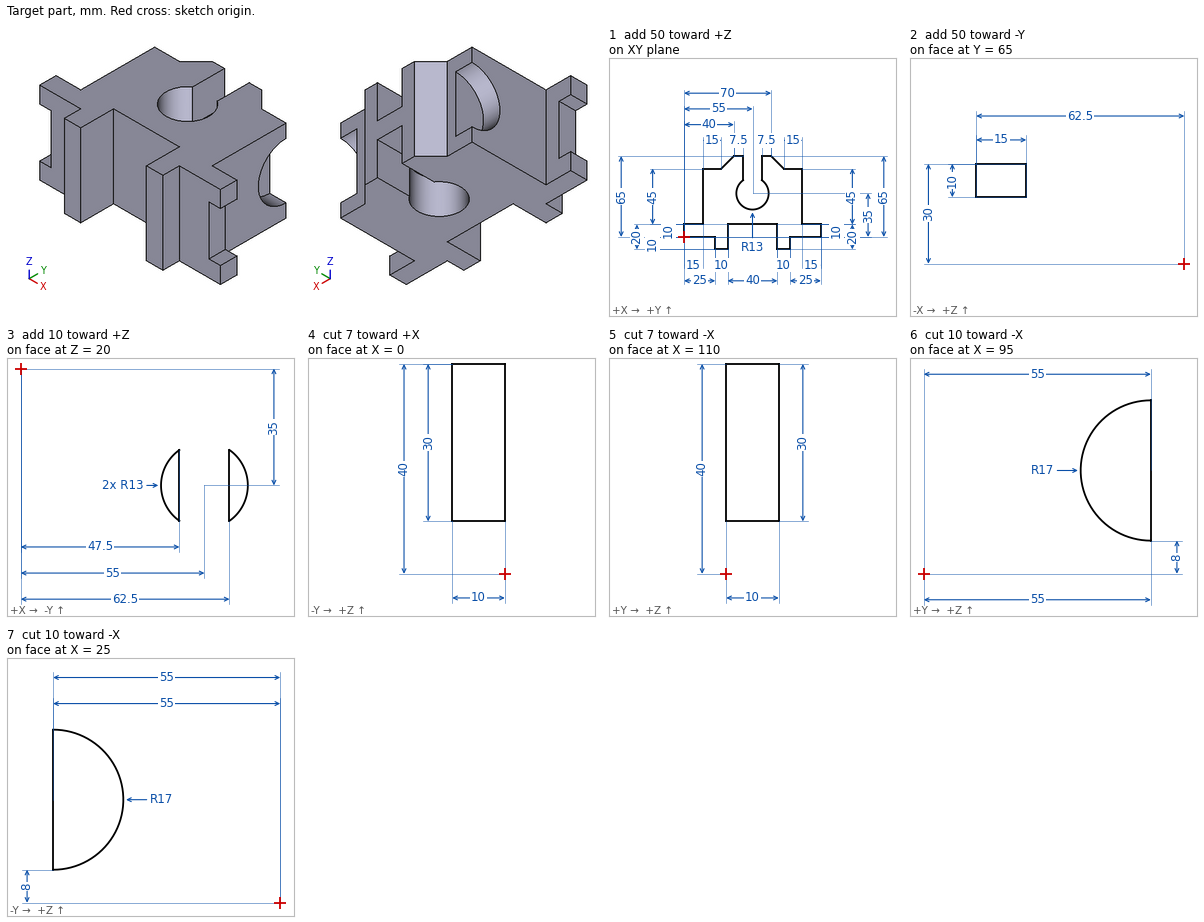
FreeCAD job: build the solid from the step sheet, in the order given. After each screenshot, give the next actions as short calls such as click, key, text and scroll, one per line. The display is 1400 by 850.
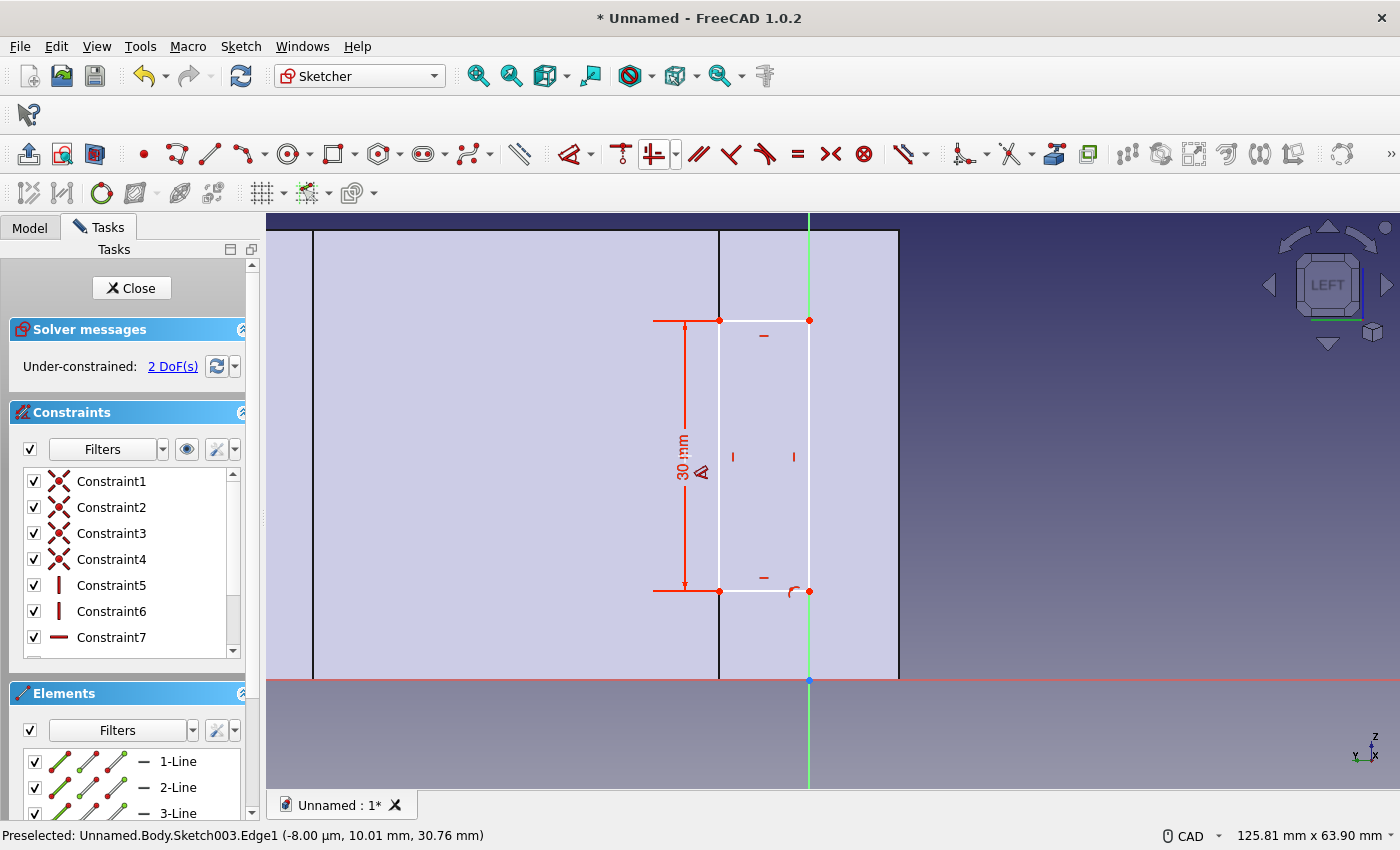
click(746, 591)
click(764, 625)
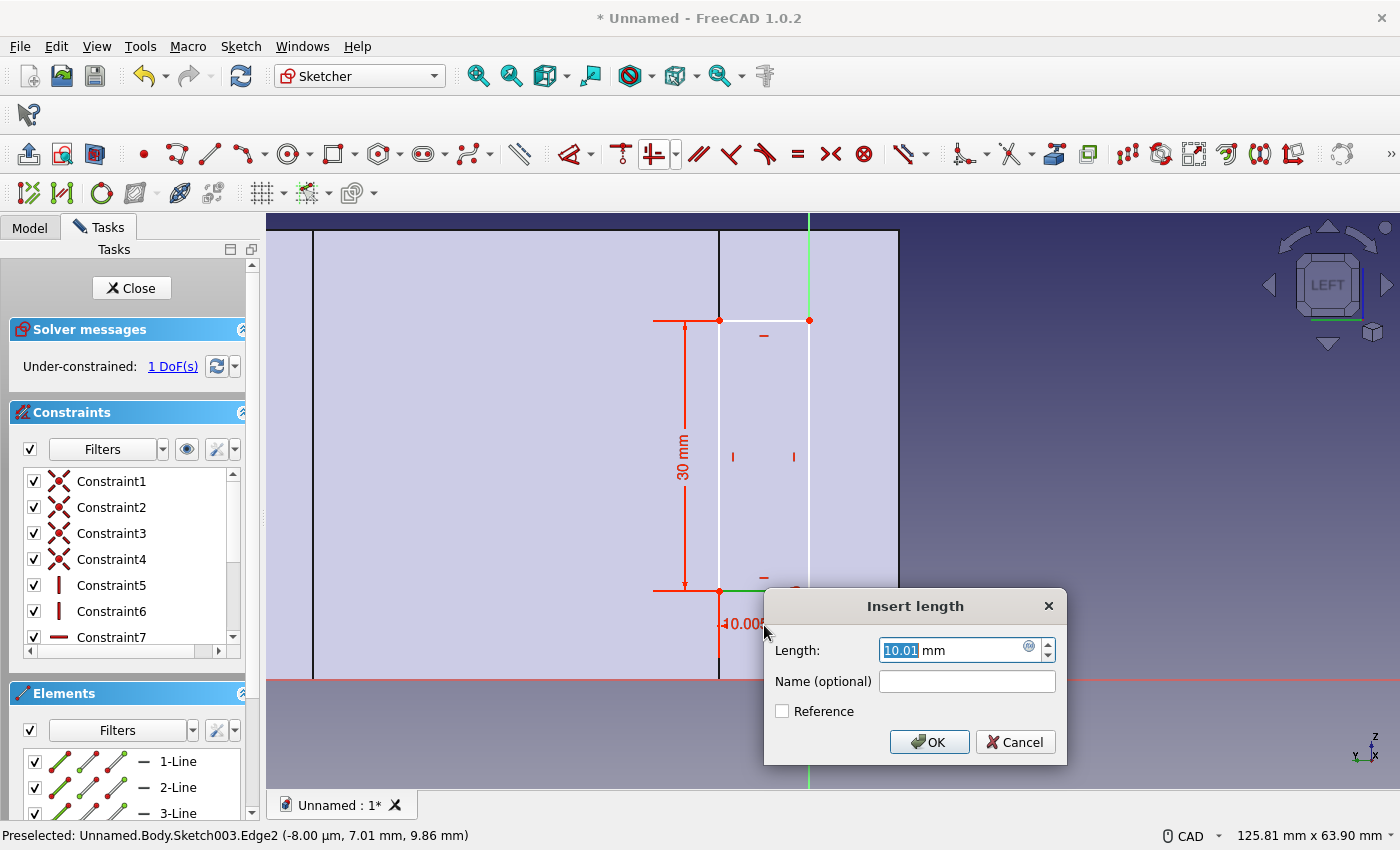
text(10)
key(Return)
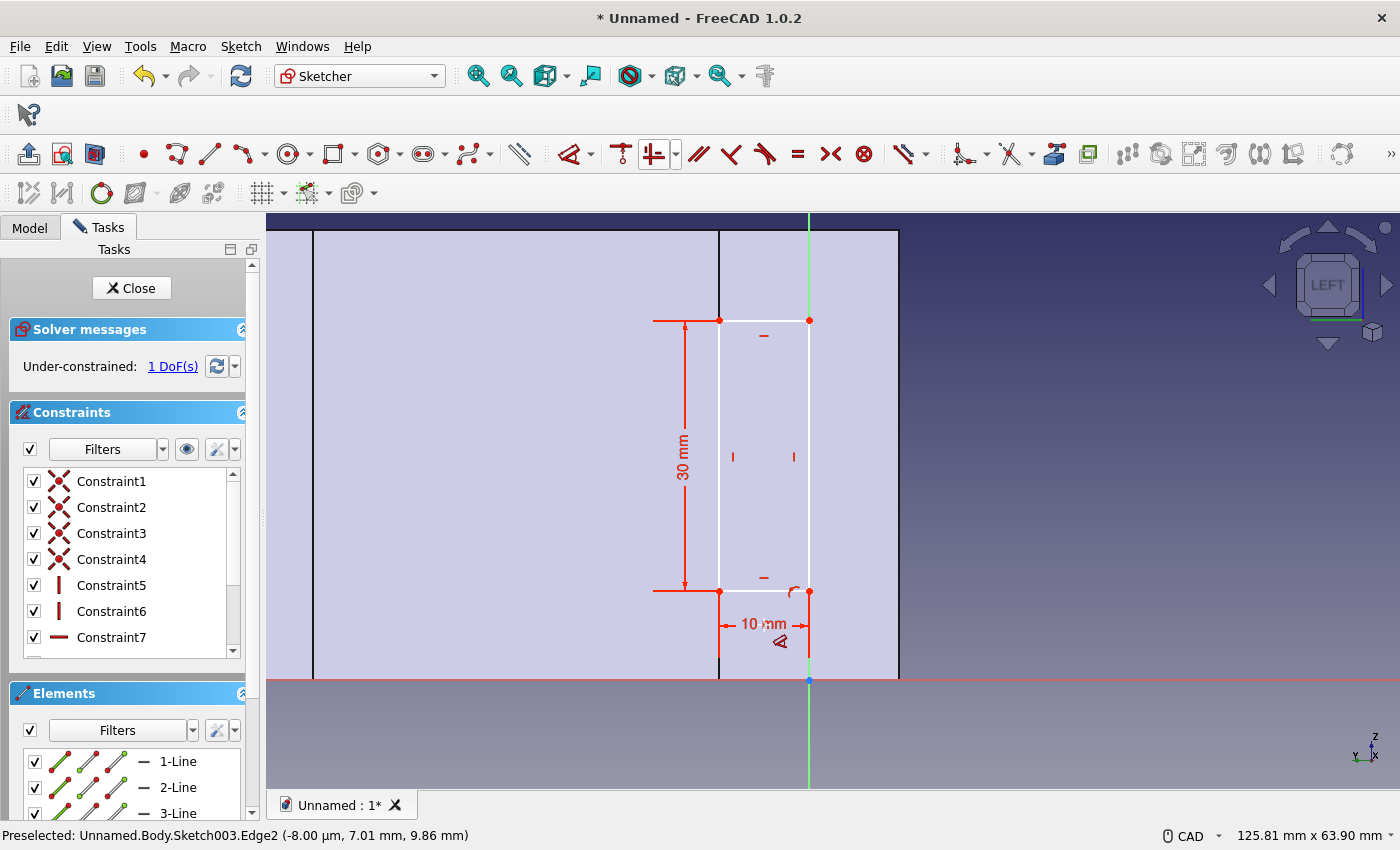
click(719, 321)
click(843, 501)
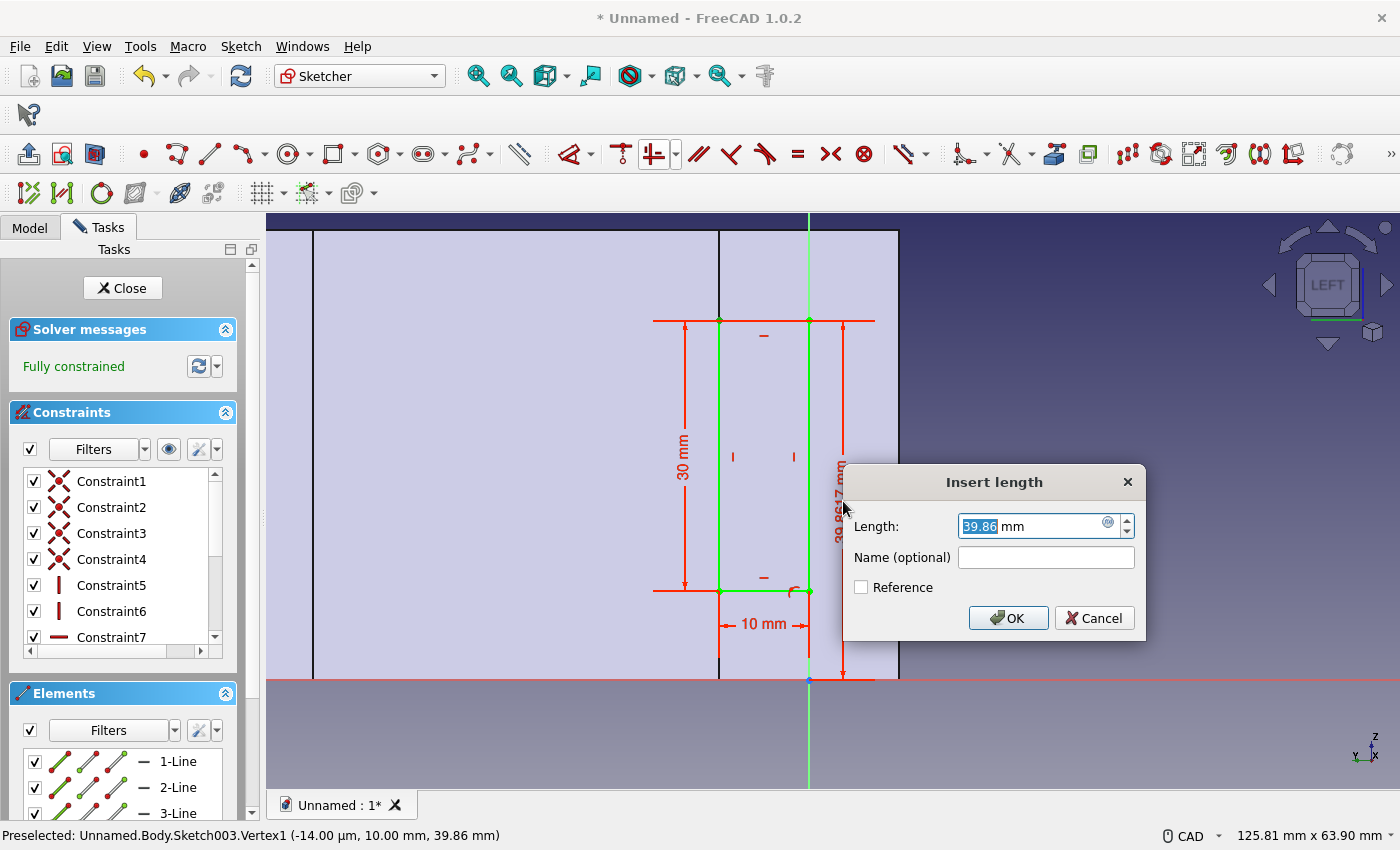
text(40)
key(Return)
key(Escape)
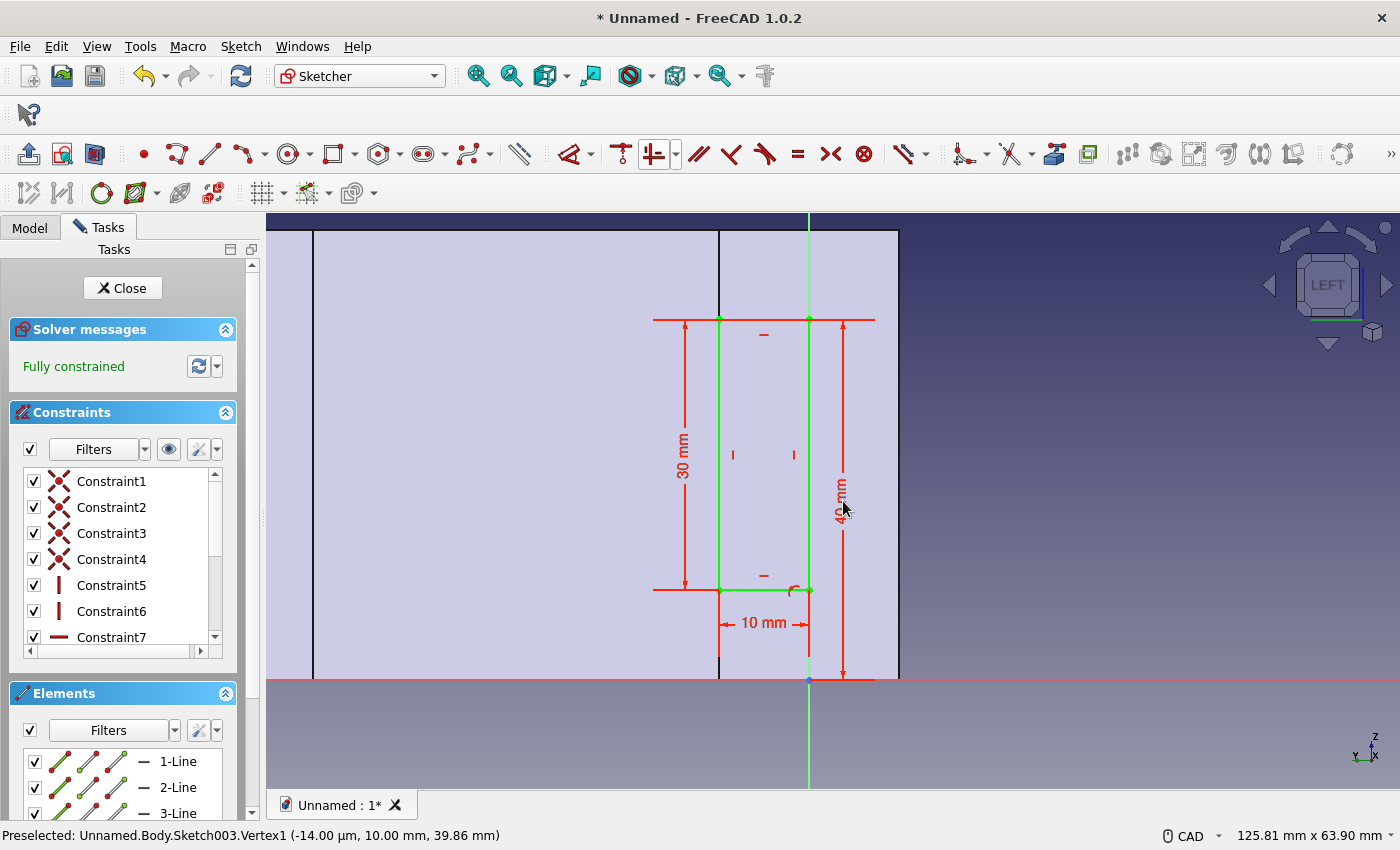
click(123, 288)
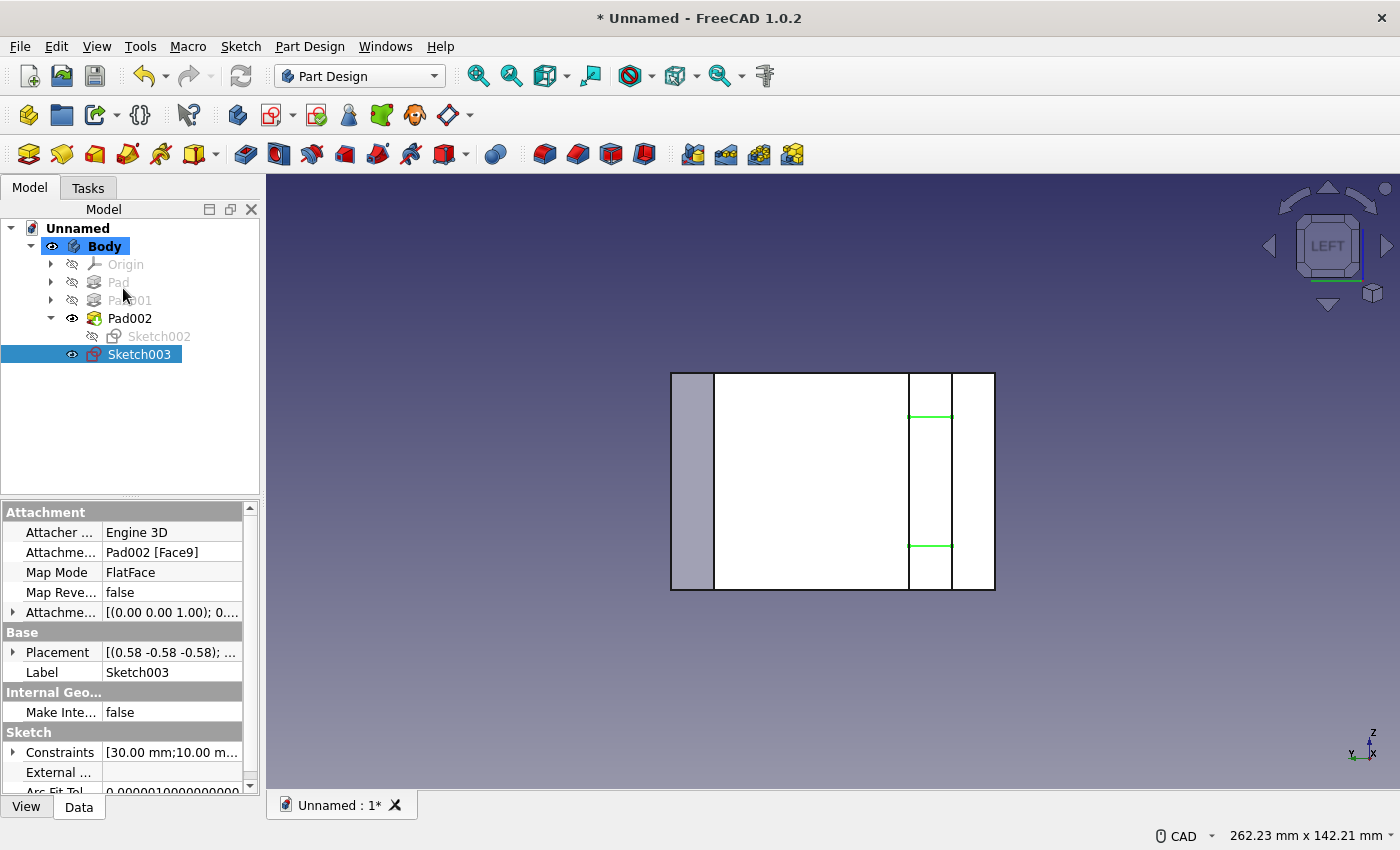
click(246, 154)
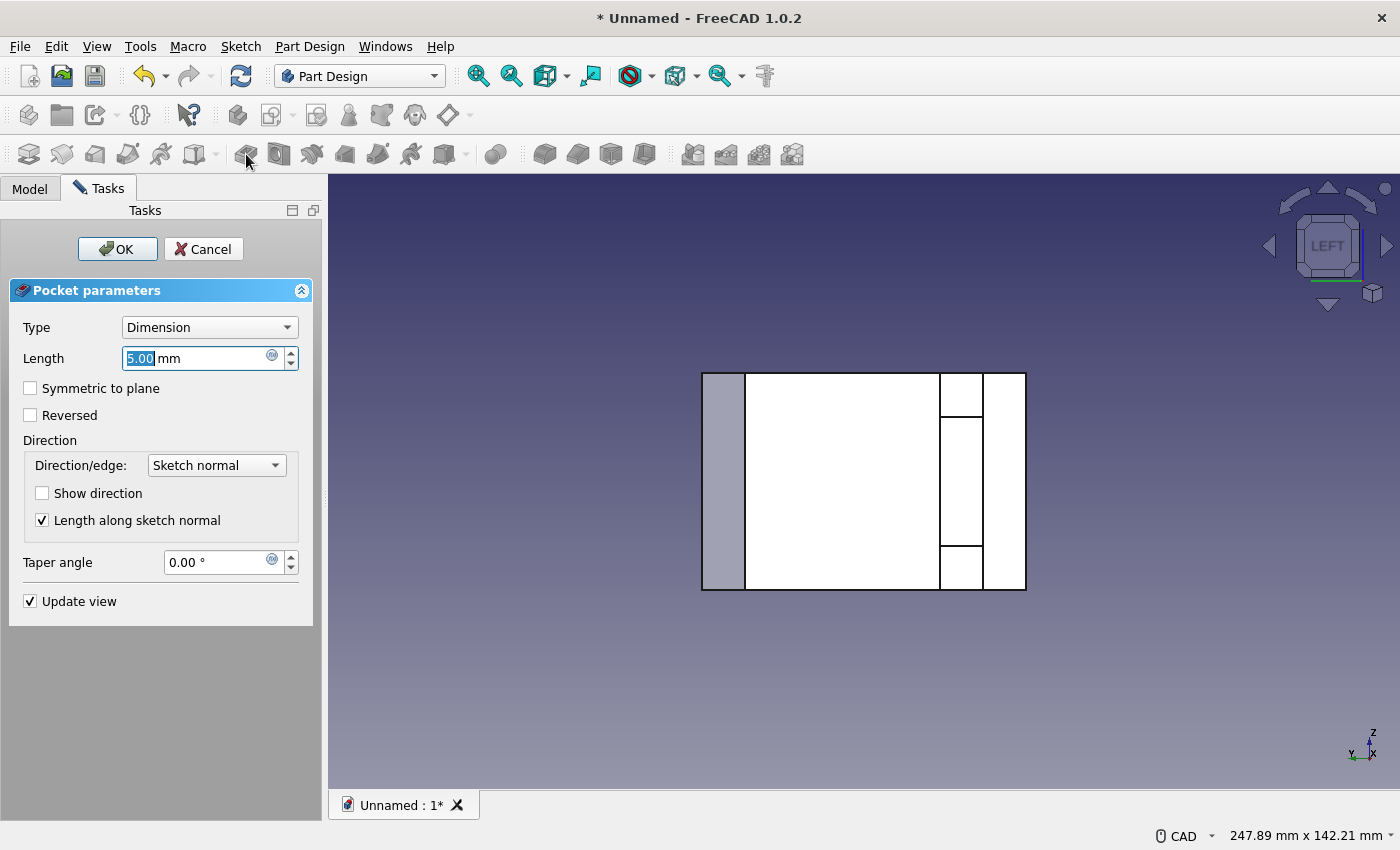
text(7)
key(Tab)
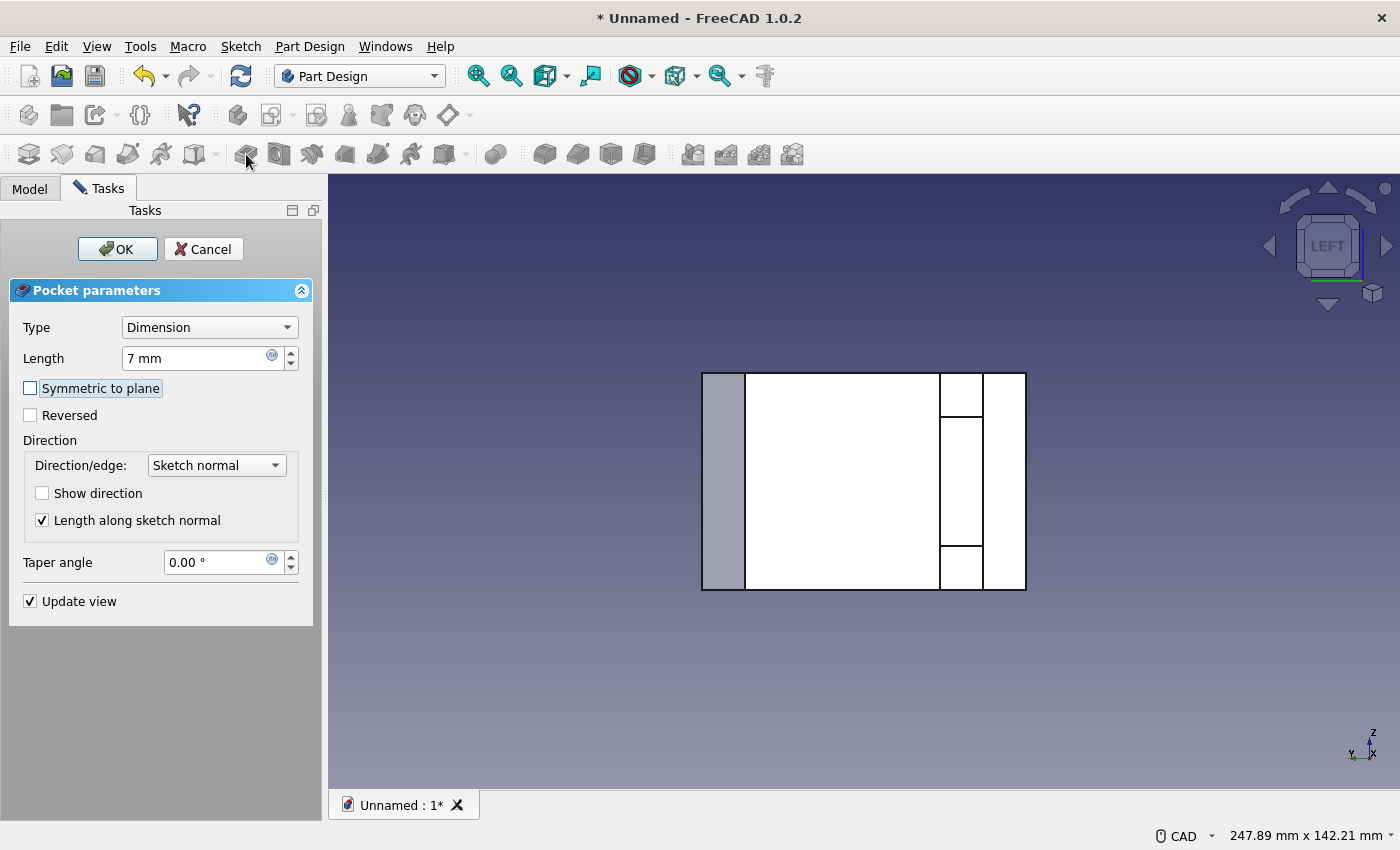
click(118, 249)